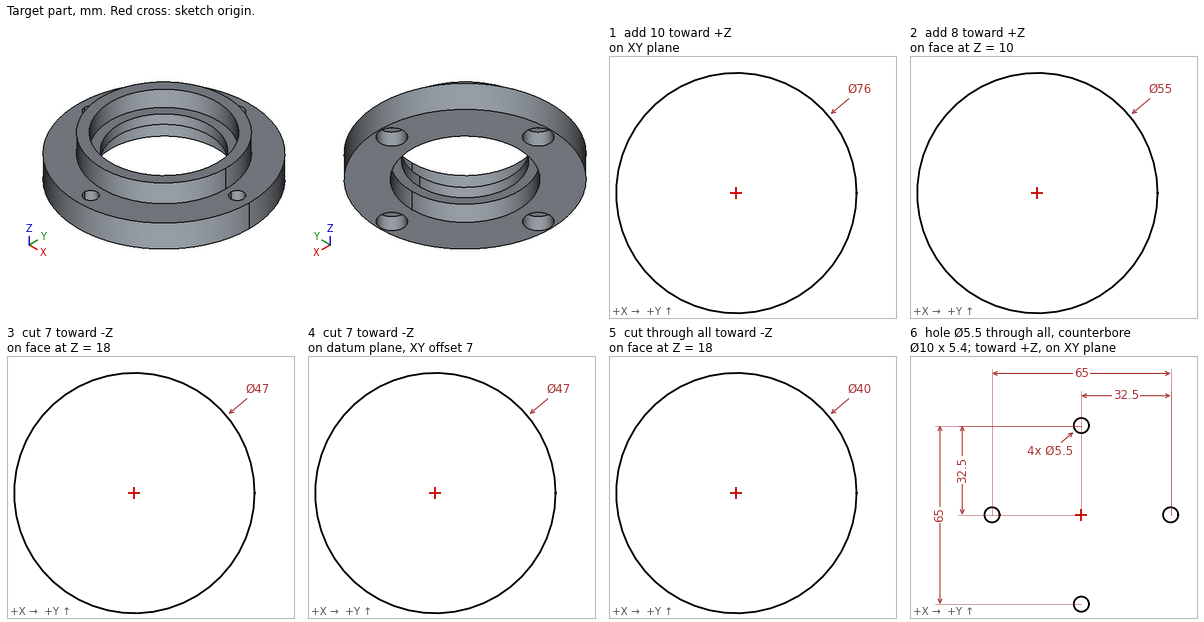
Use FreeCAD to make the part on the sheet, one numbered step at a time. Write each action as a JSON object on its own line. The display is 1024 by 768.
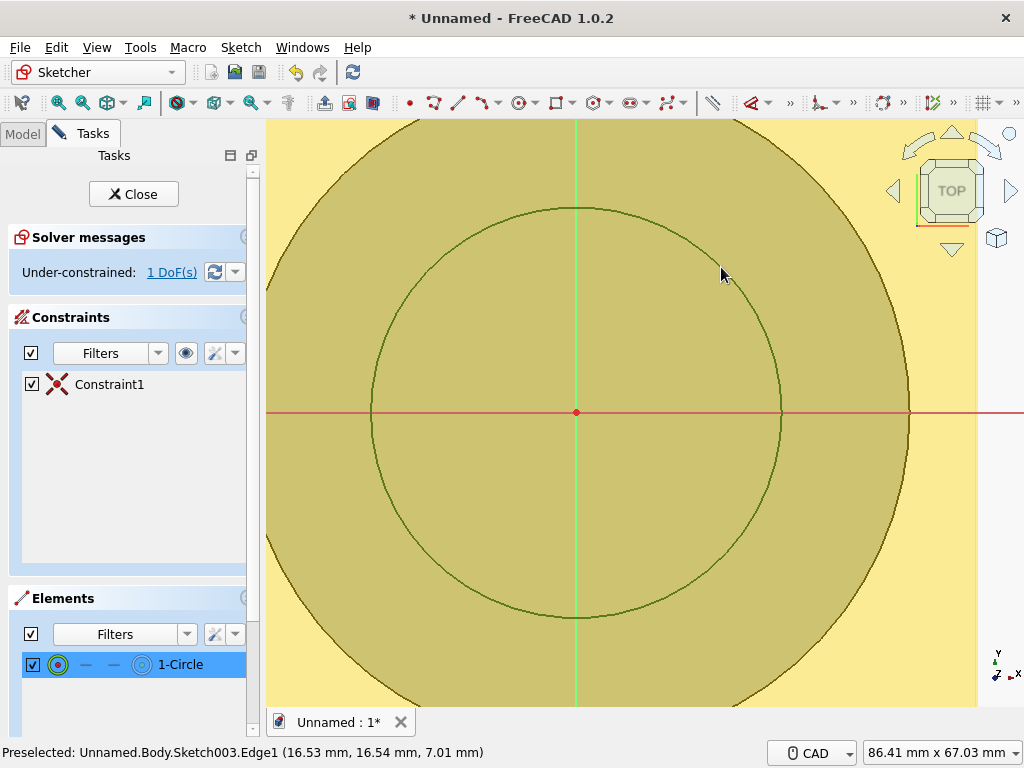
{"action": "key", "text": "k o"}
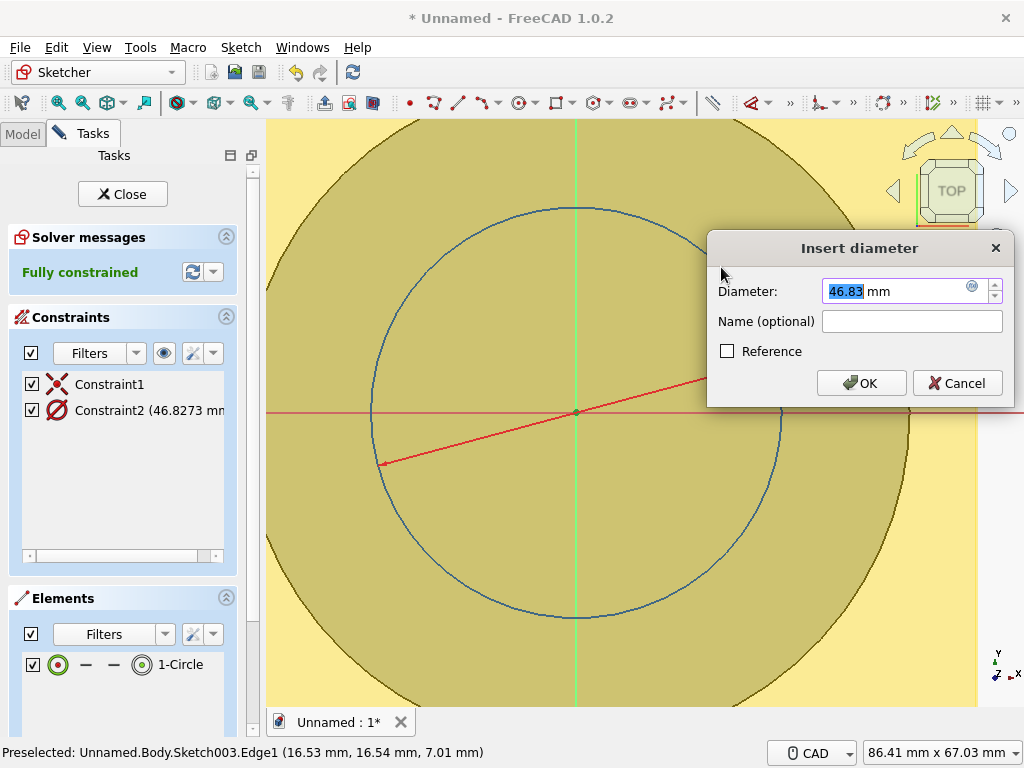
{"action": "type", "text": "47"}
{"action": "key", "text": "Return"}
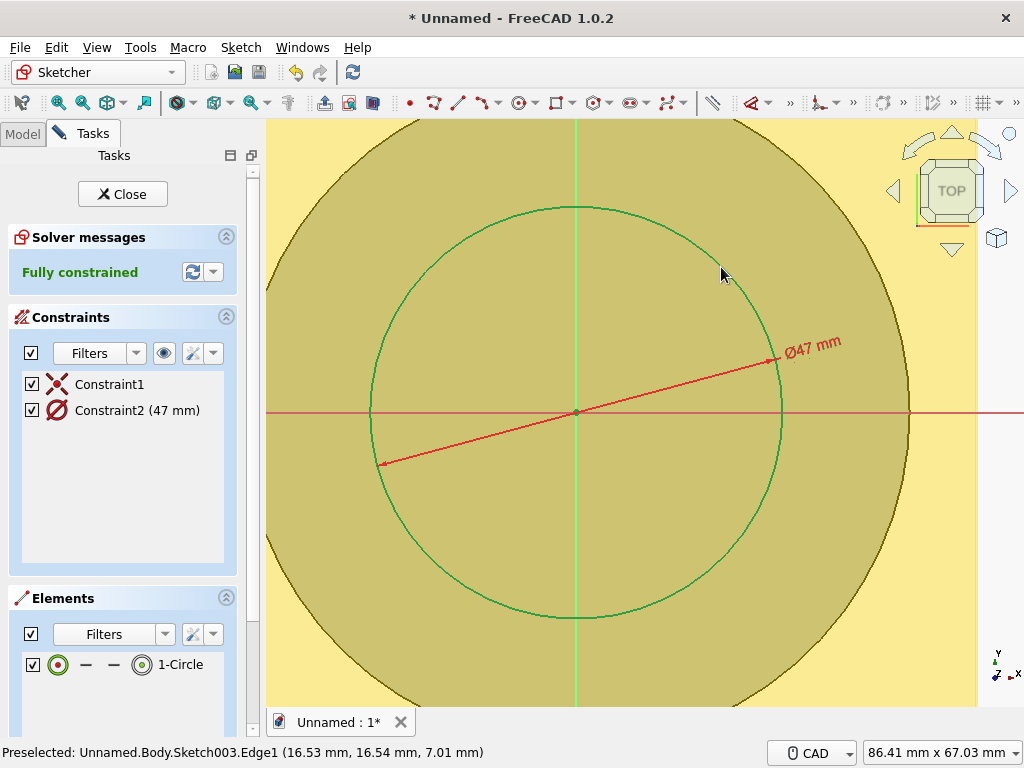
{"action": "left_click", "coordinate": [123, 194]}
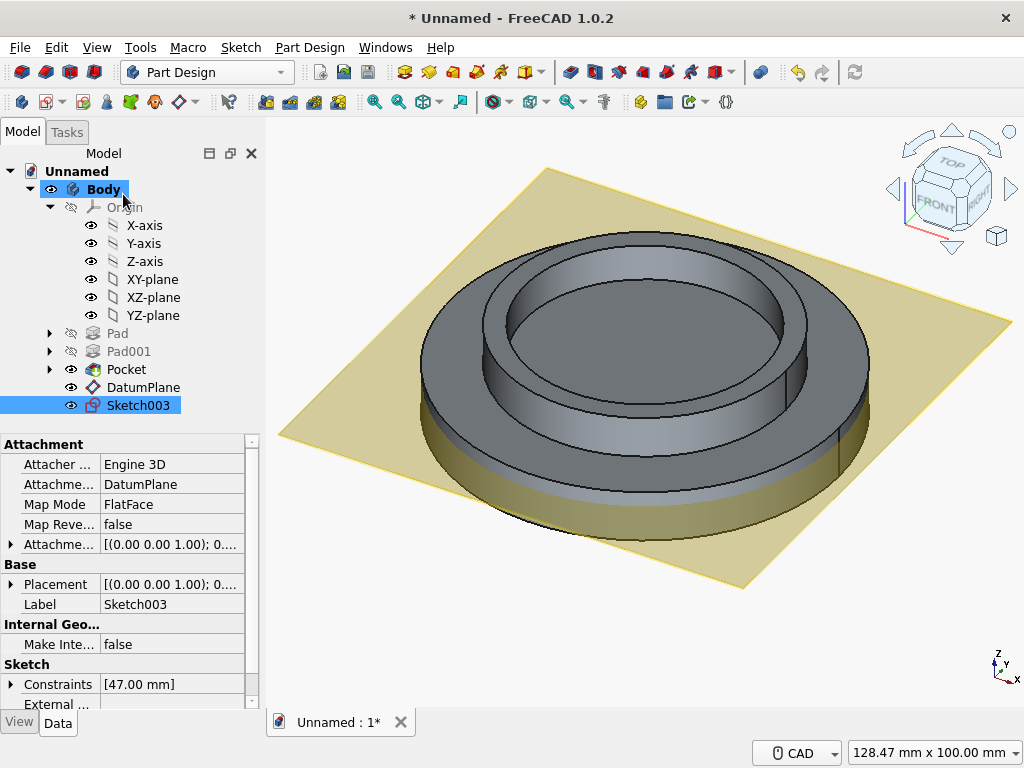
{"action": "left_click", "coordinate": [572, 72]}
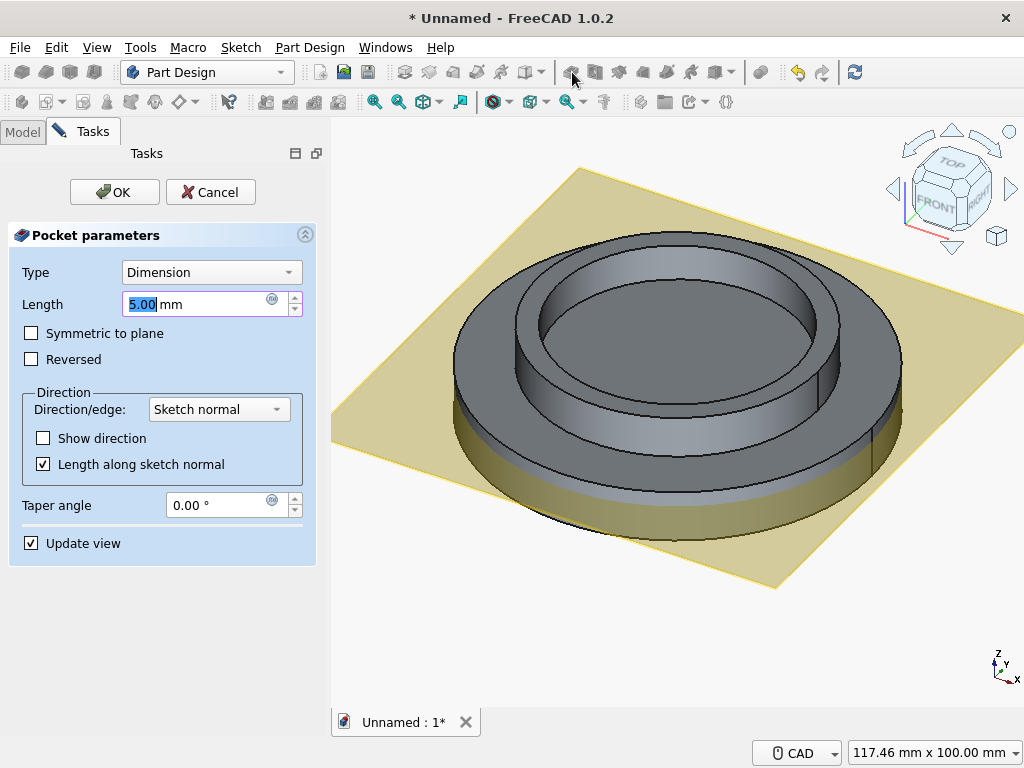
{"action": "type", "text": "7"}
{"action": "key", "text": "Tab"}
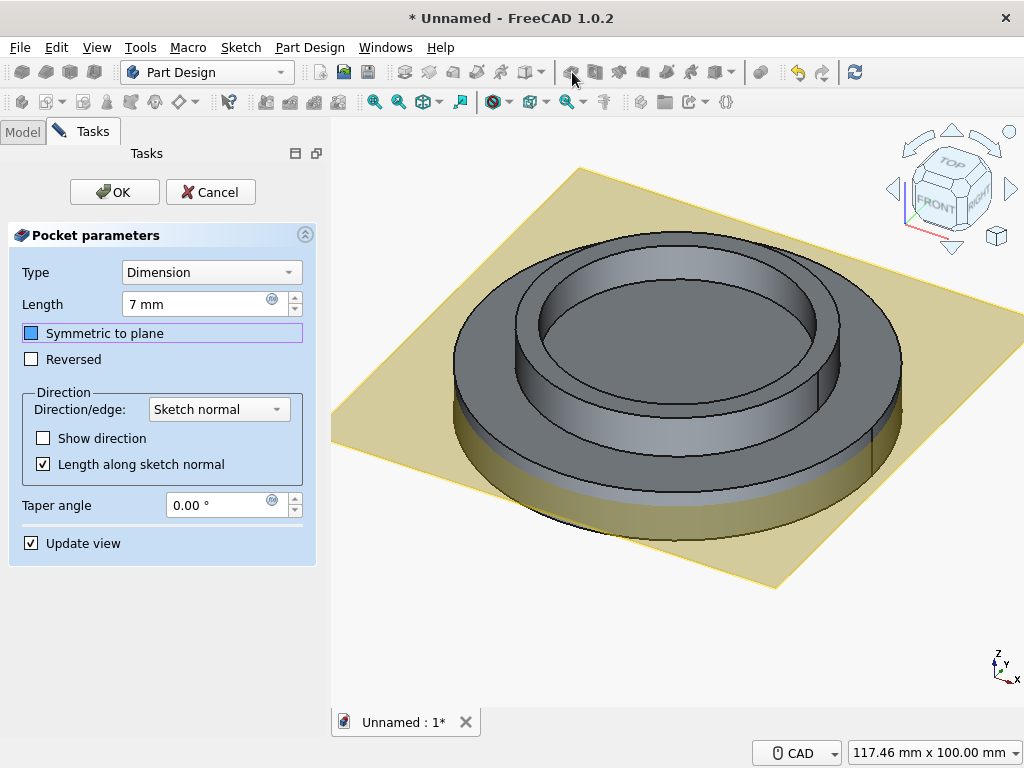
{"action": "left_click", "coordinate": [115, 192]}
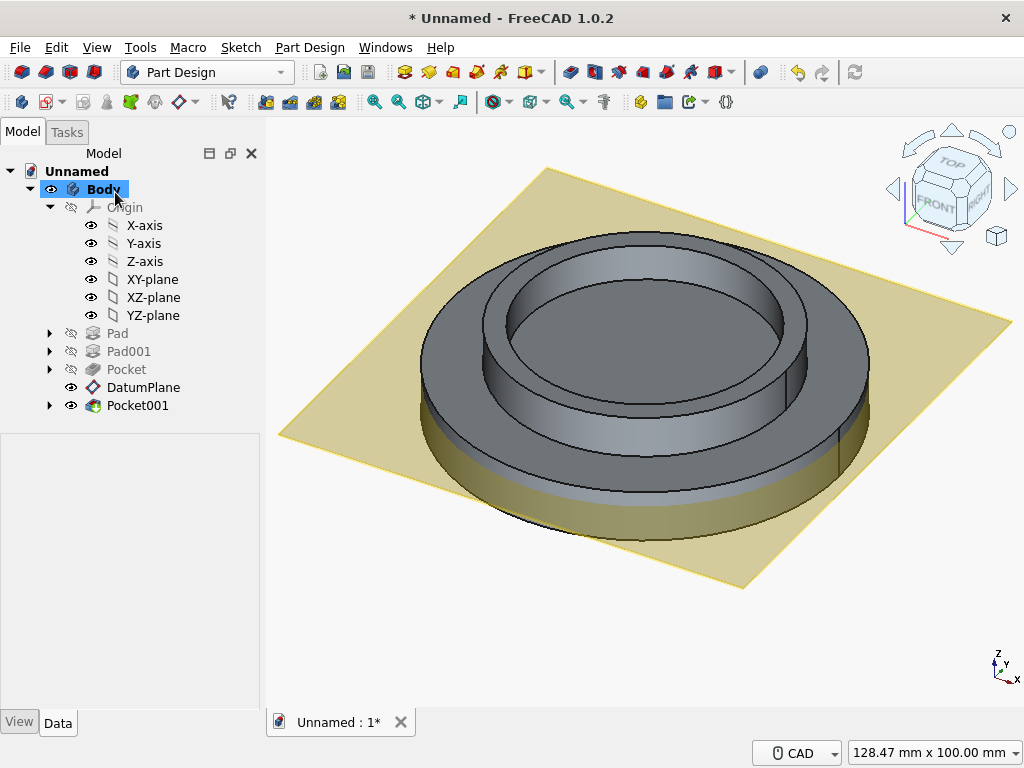
{"action": "left_click", "coordinate": [116, 387]}
{"action": "key", "text": "space"}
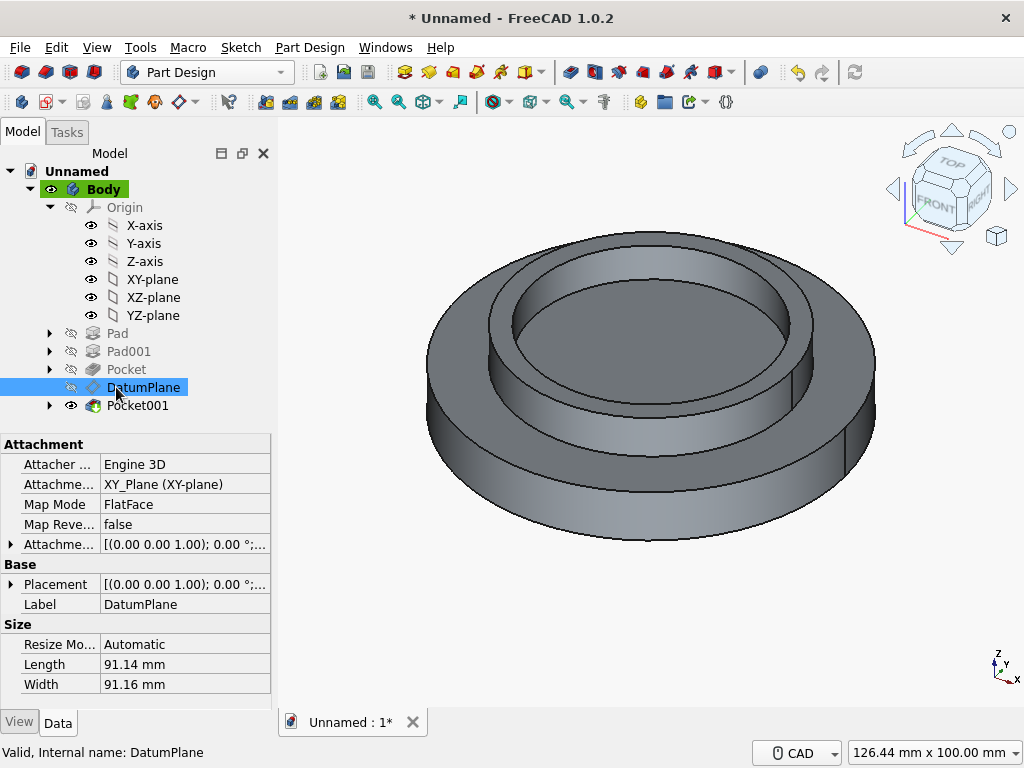
{"action": "left_click", "coordinate": [541, 380]}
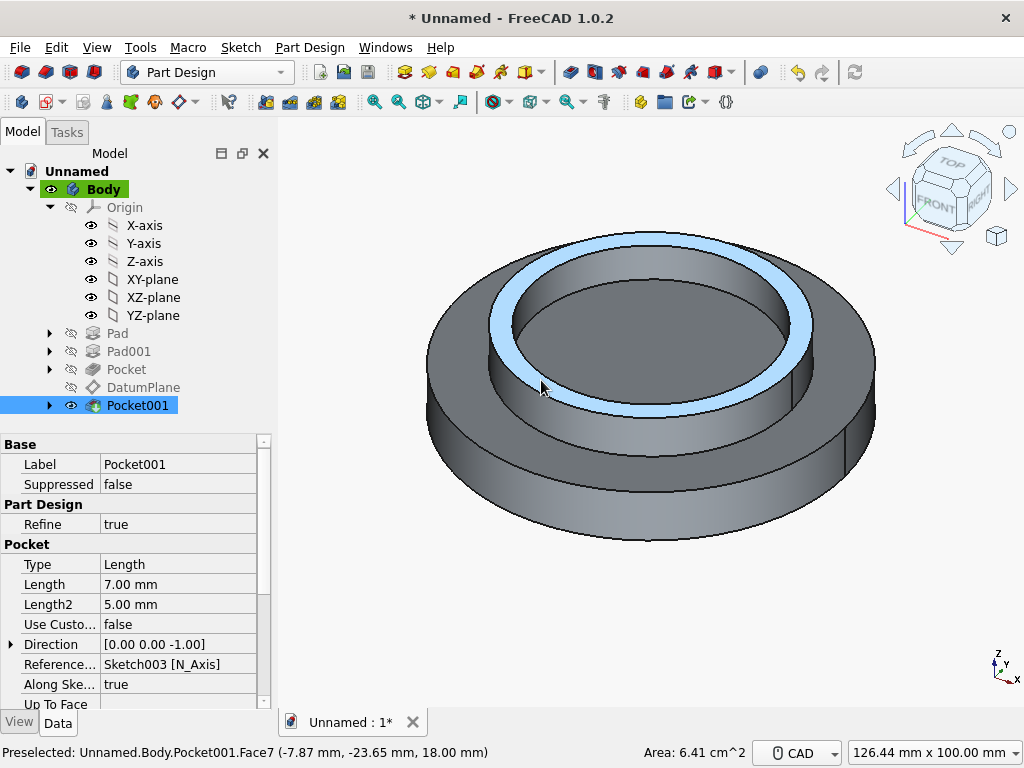
{"action": "left_click", "coordinate": [46, 102]}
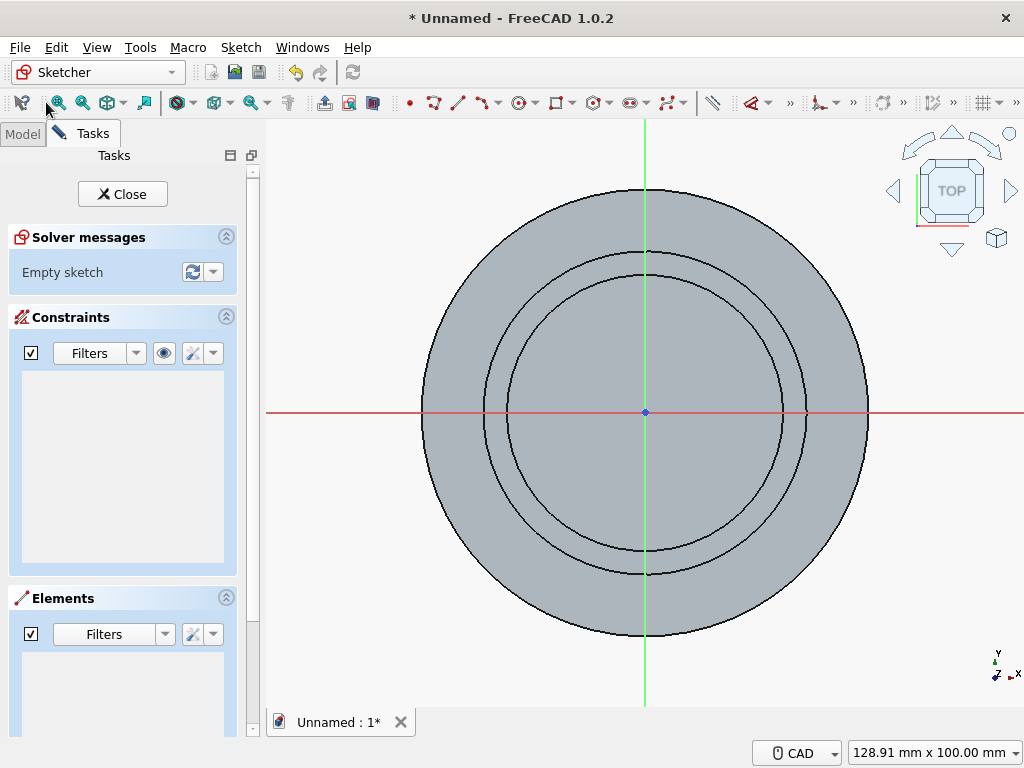
{"action": "scroll", "coordinate": [784, 413], "scroll_direction": "up", "scroll_amount": 2}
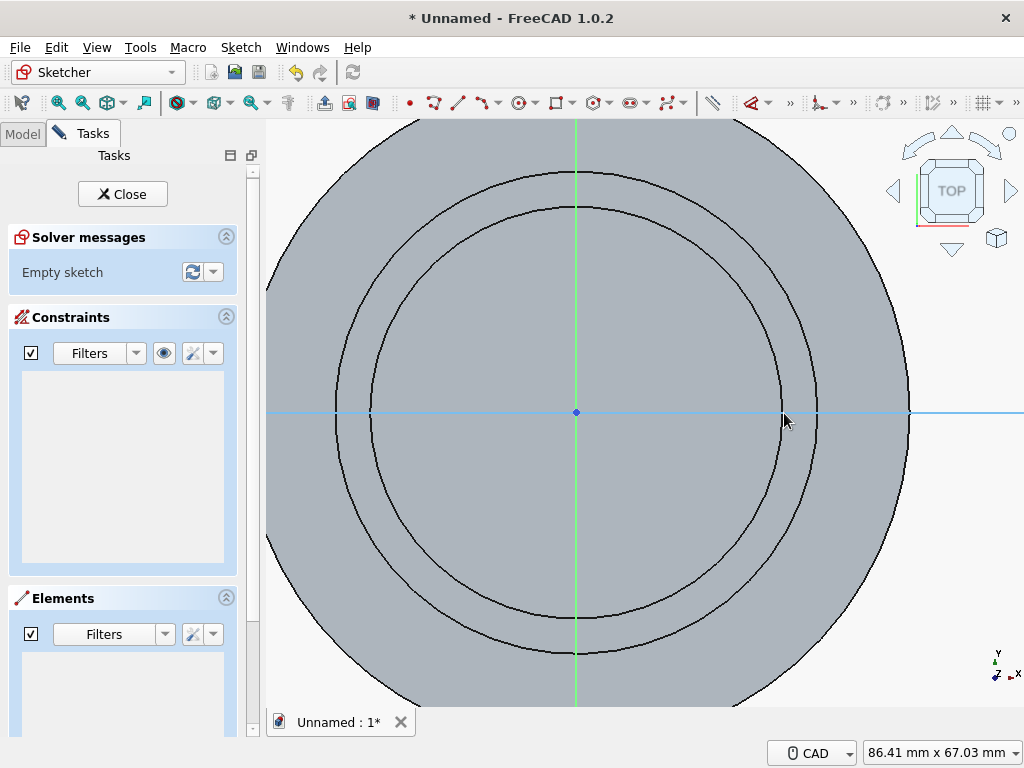
{"action": "key", "text": "g c"}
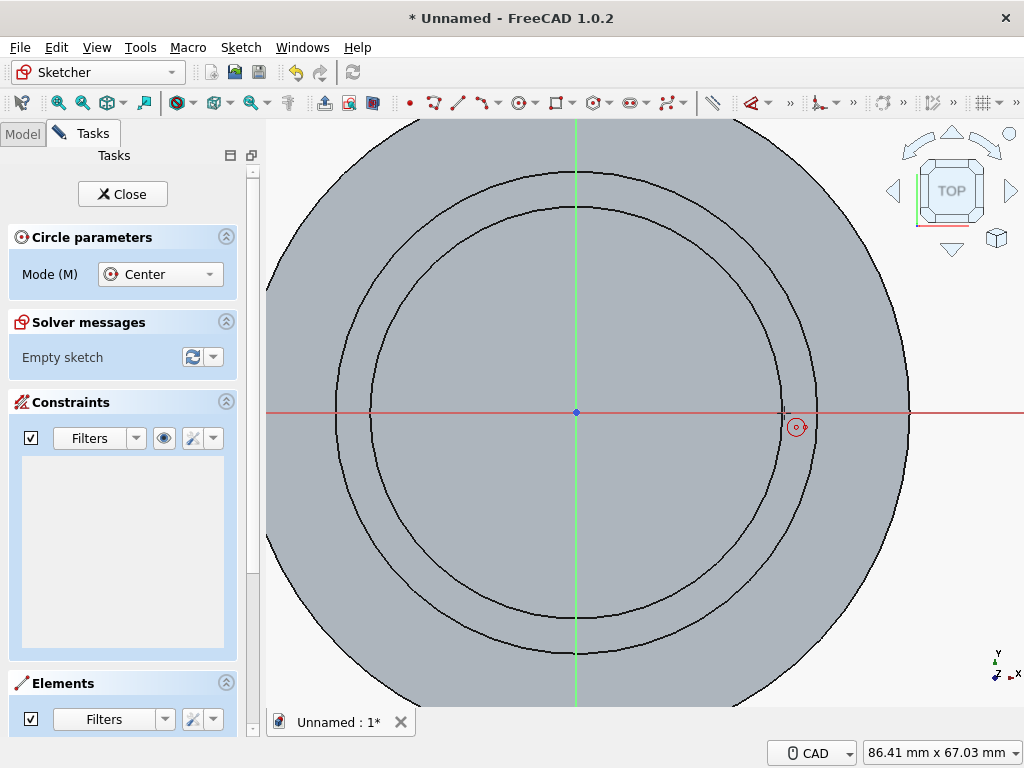
{"action": "left_click", "coordinate": [576, 413]}
{"action": "left_click", "coordinate": [700, 289]}
{"action": "key", "text": "Escape"}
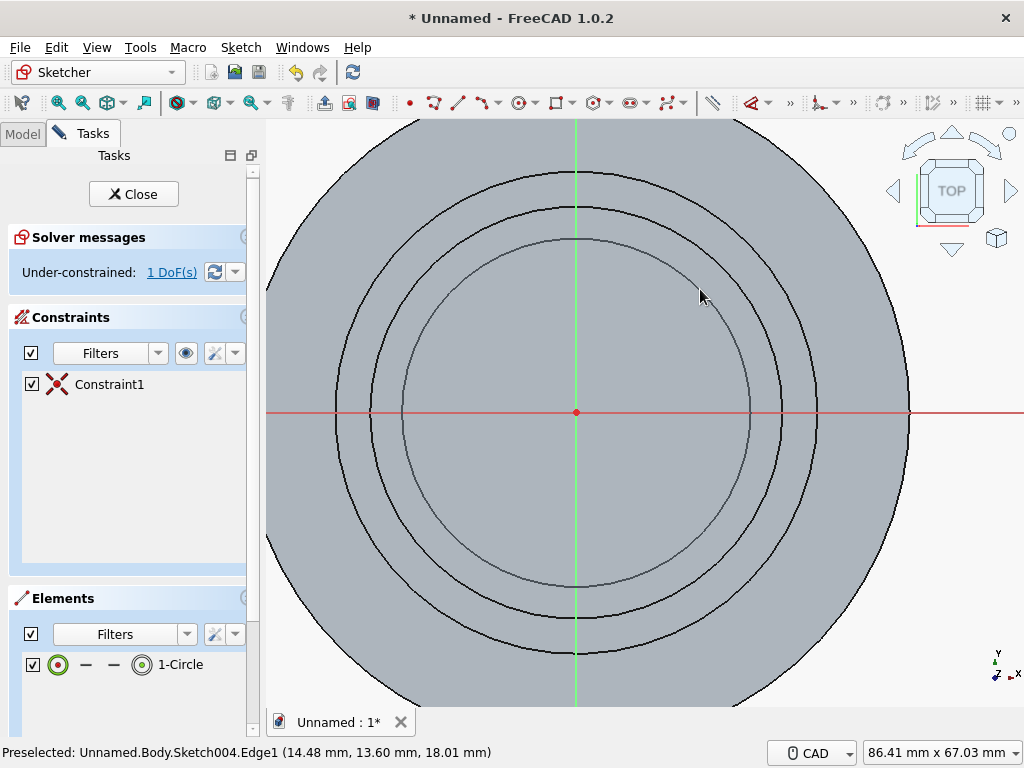
{"action": "left_click", "coordinate": [699, 289]}